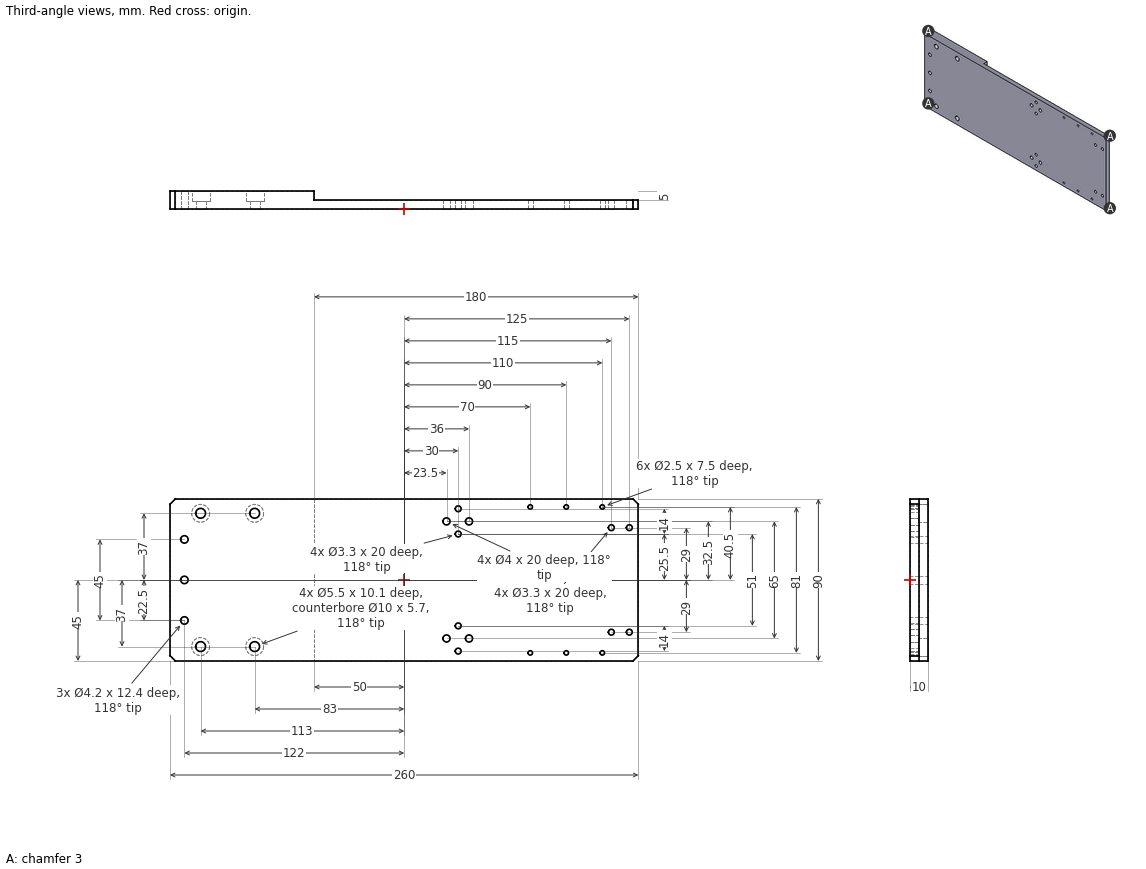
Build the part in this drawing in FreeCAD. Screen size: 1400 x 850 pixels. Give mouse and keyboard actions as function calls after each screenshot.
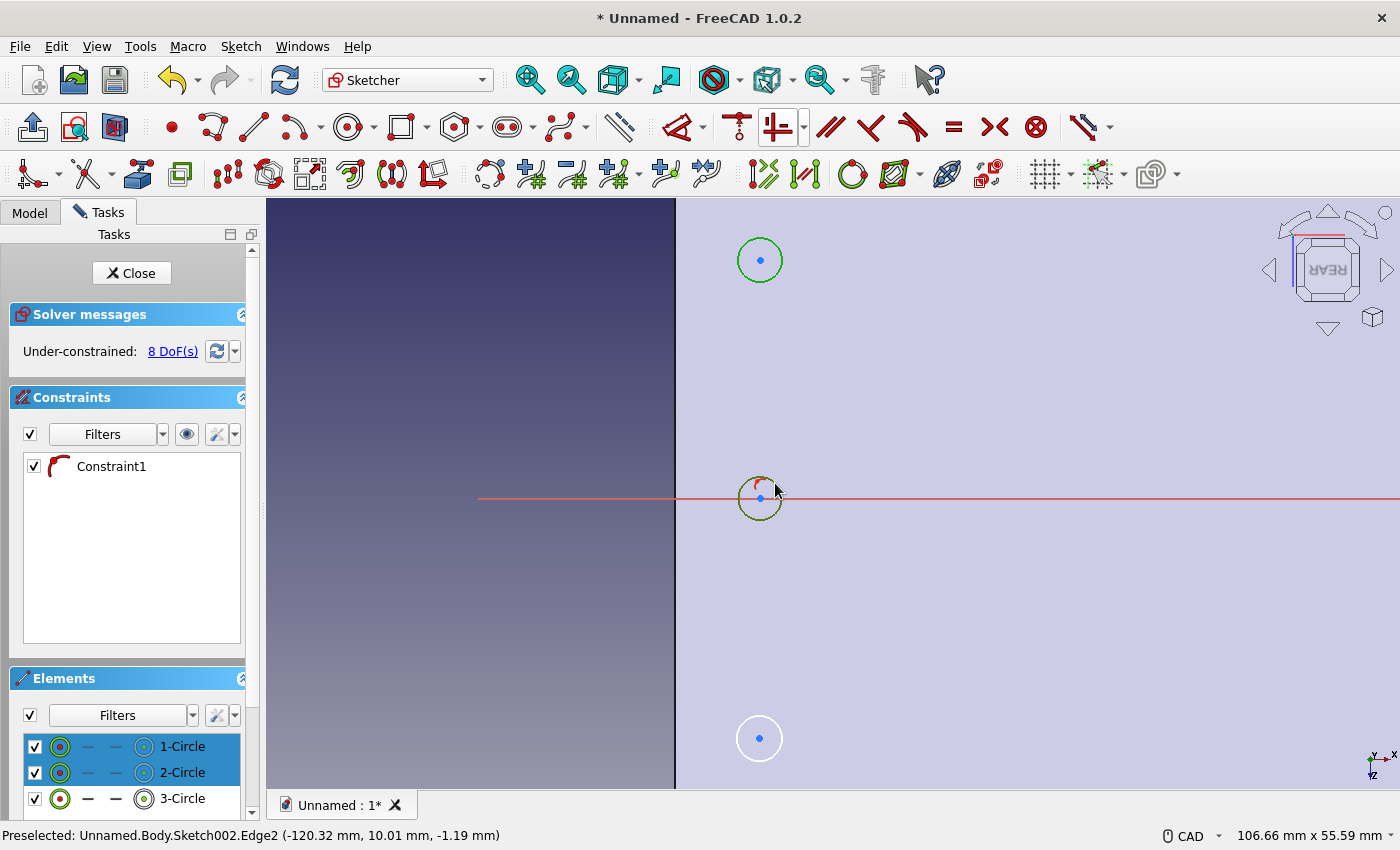
click(775, 723)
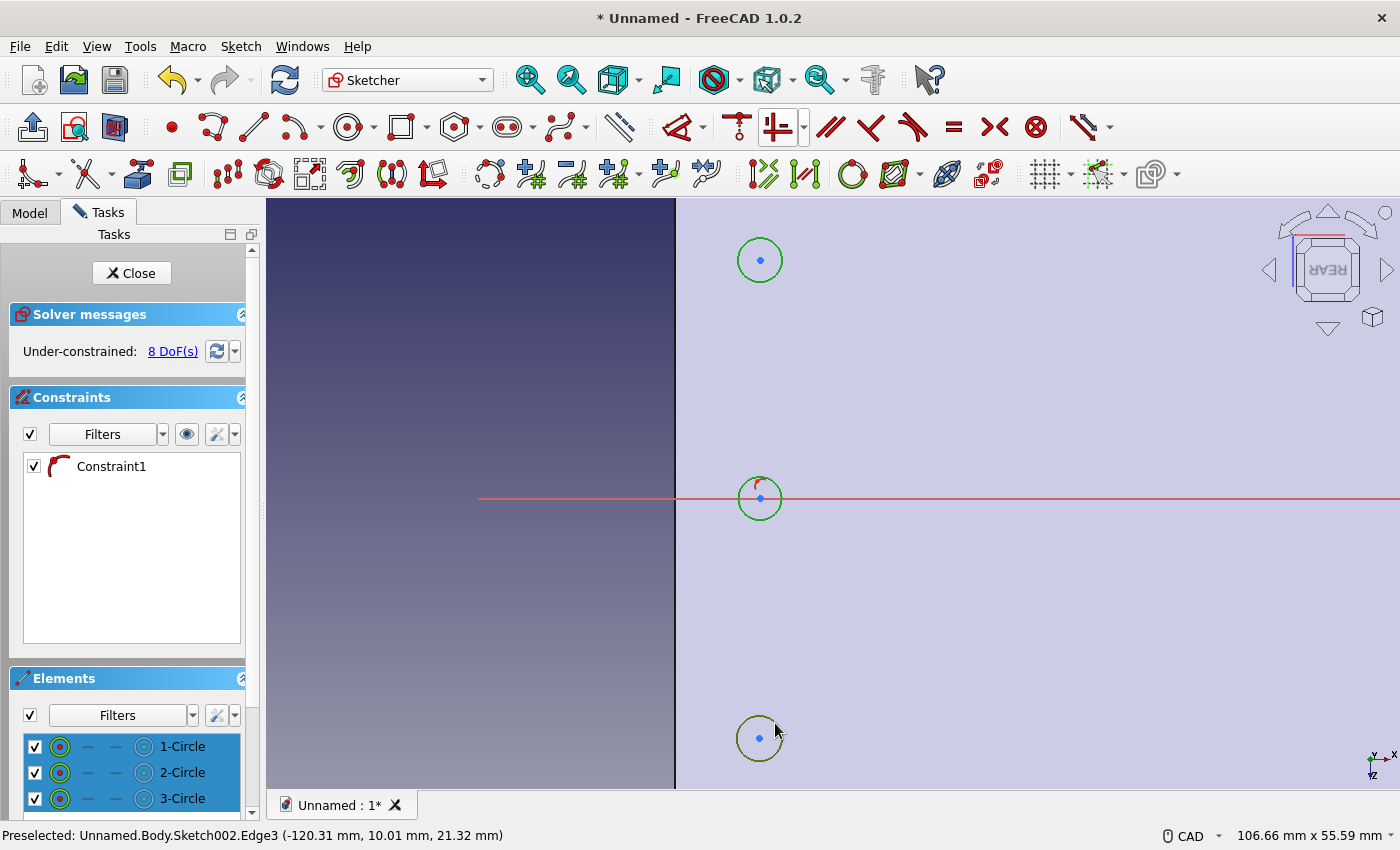
click(954, 128)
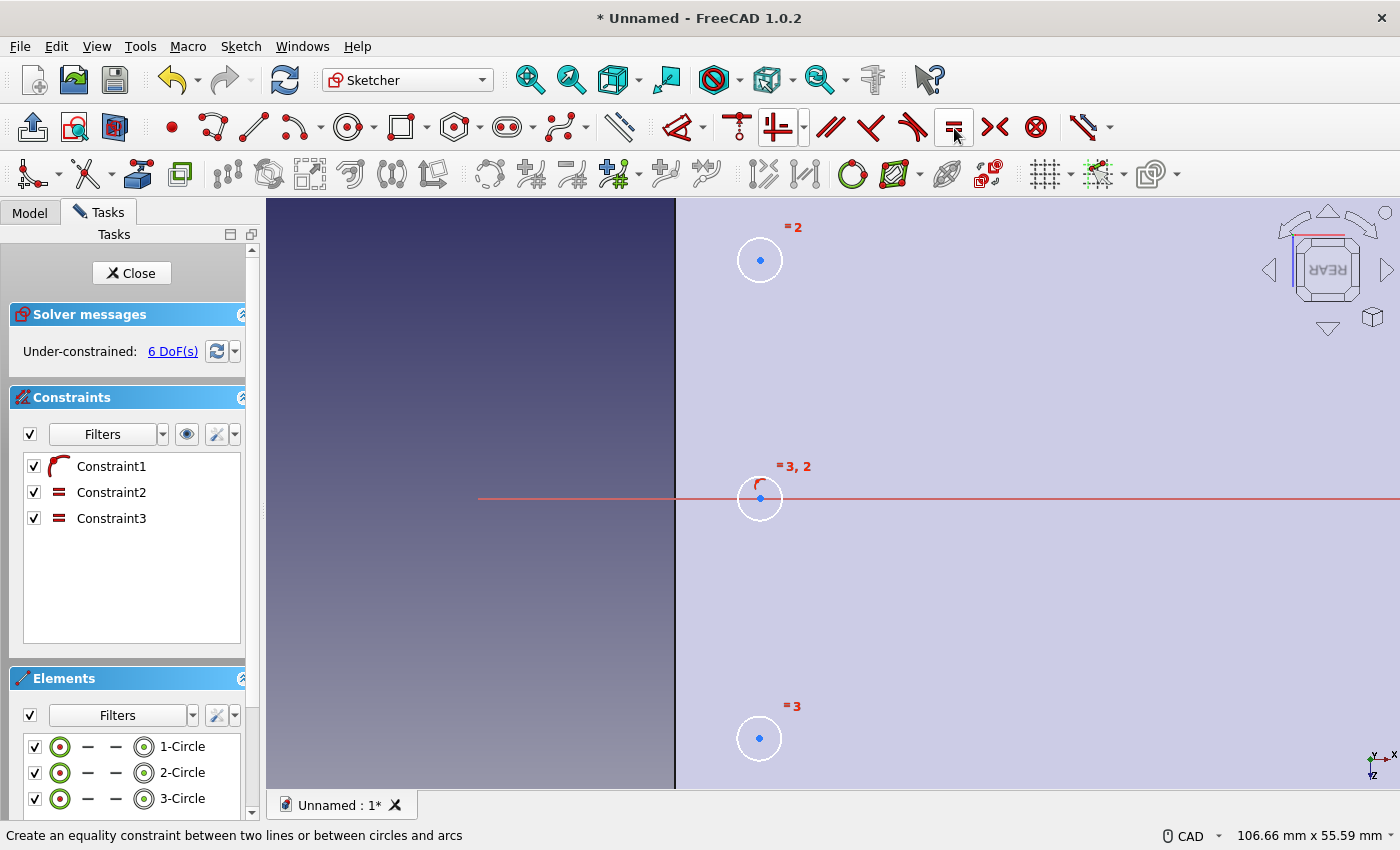
click(760, 260)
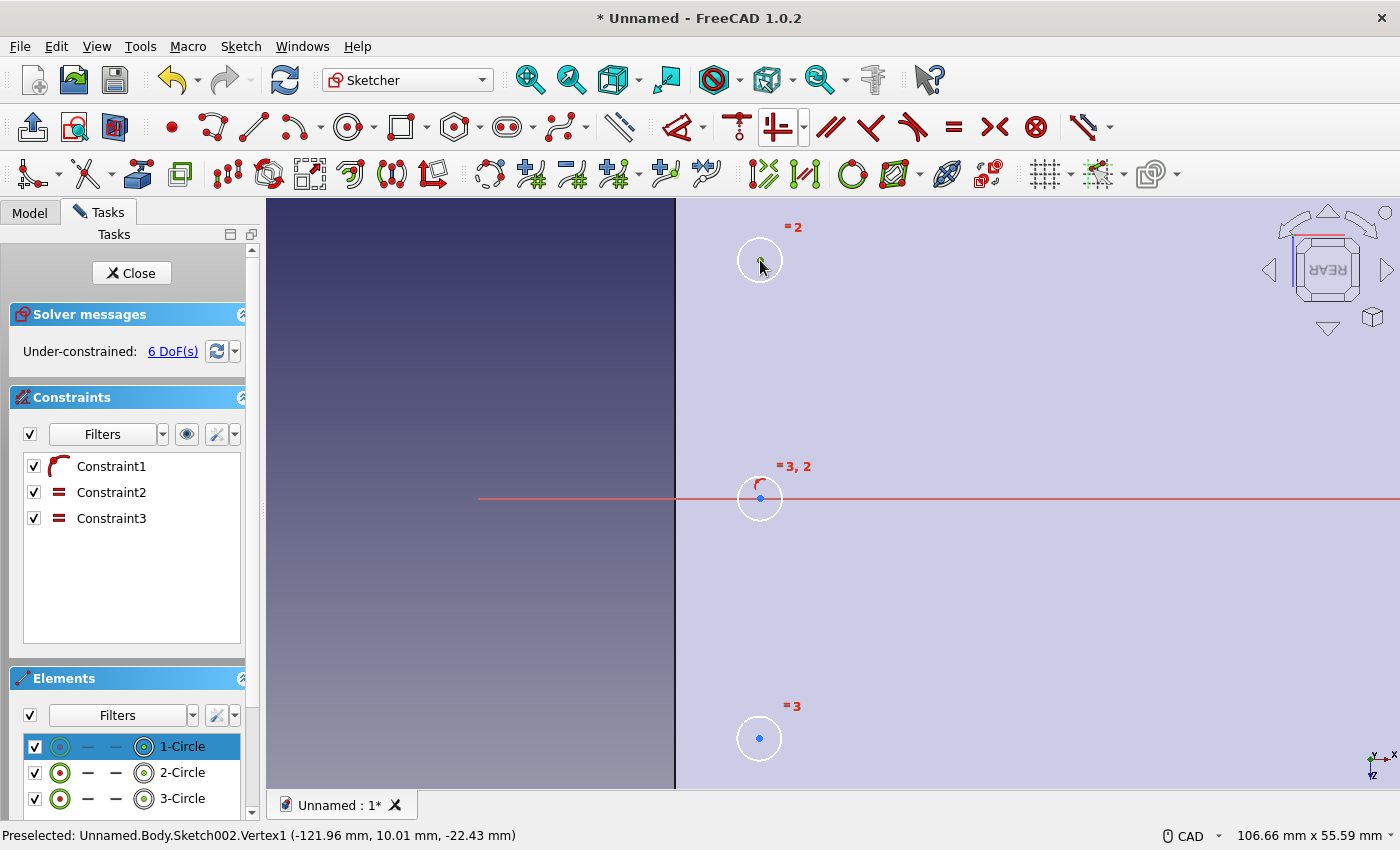
click(760, 499)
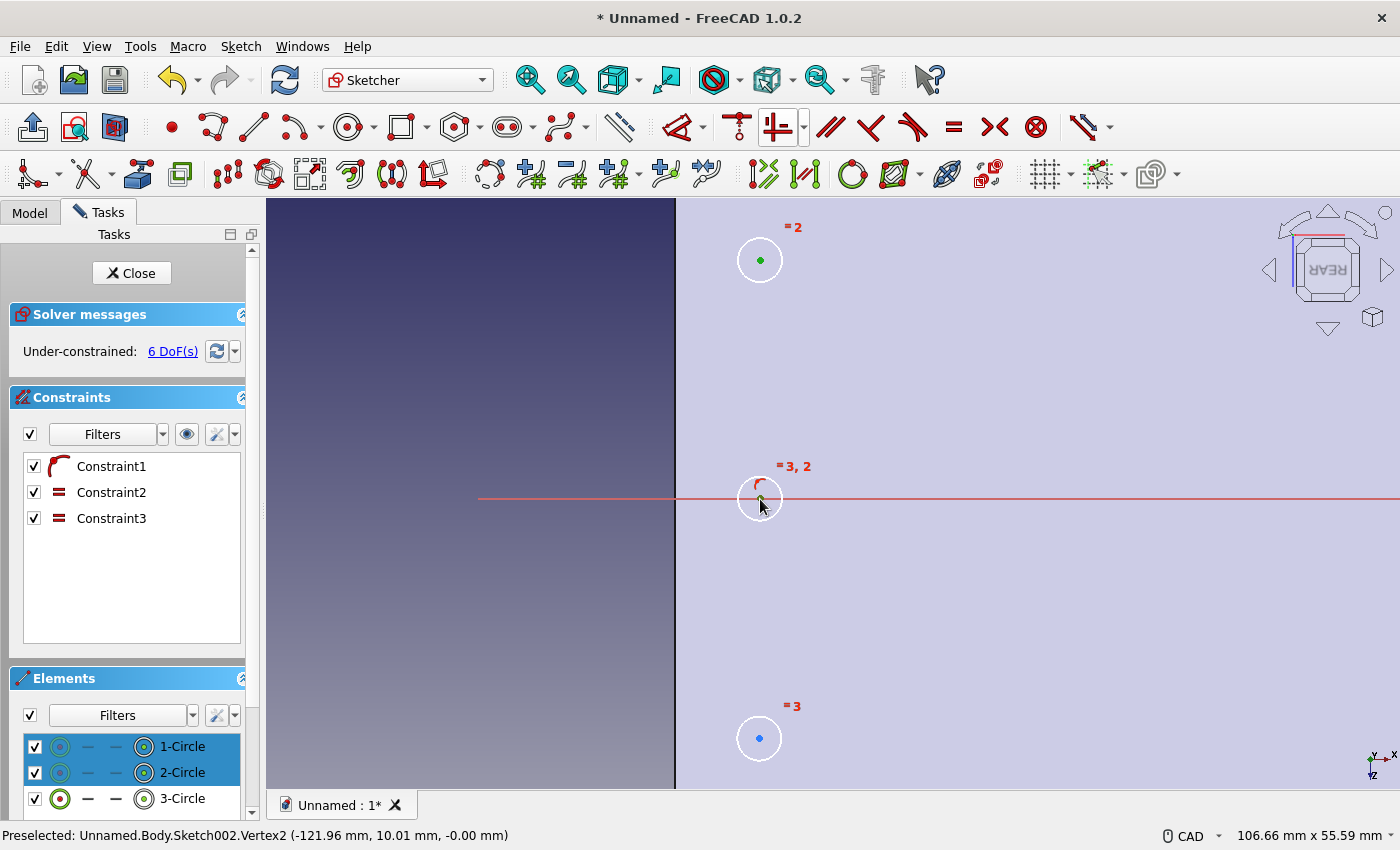
key(v)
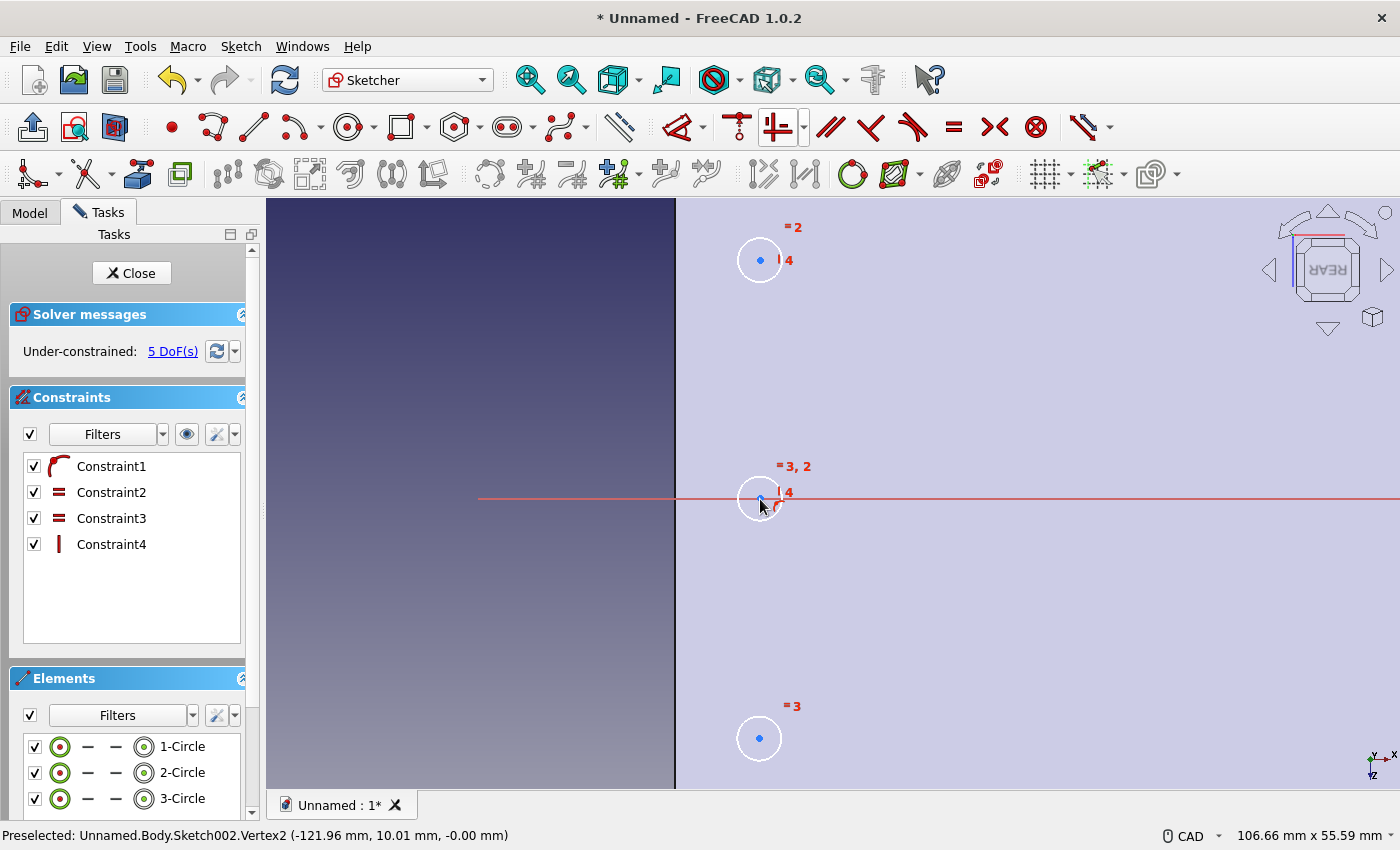
click(760, 499)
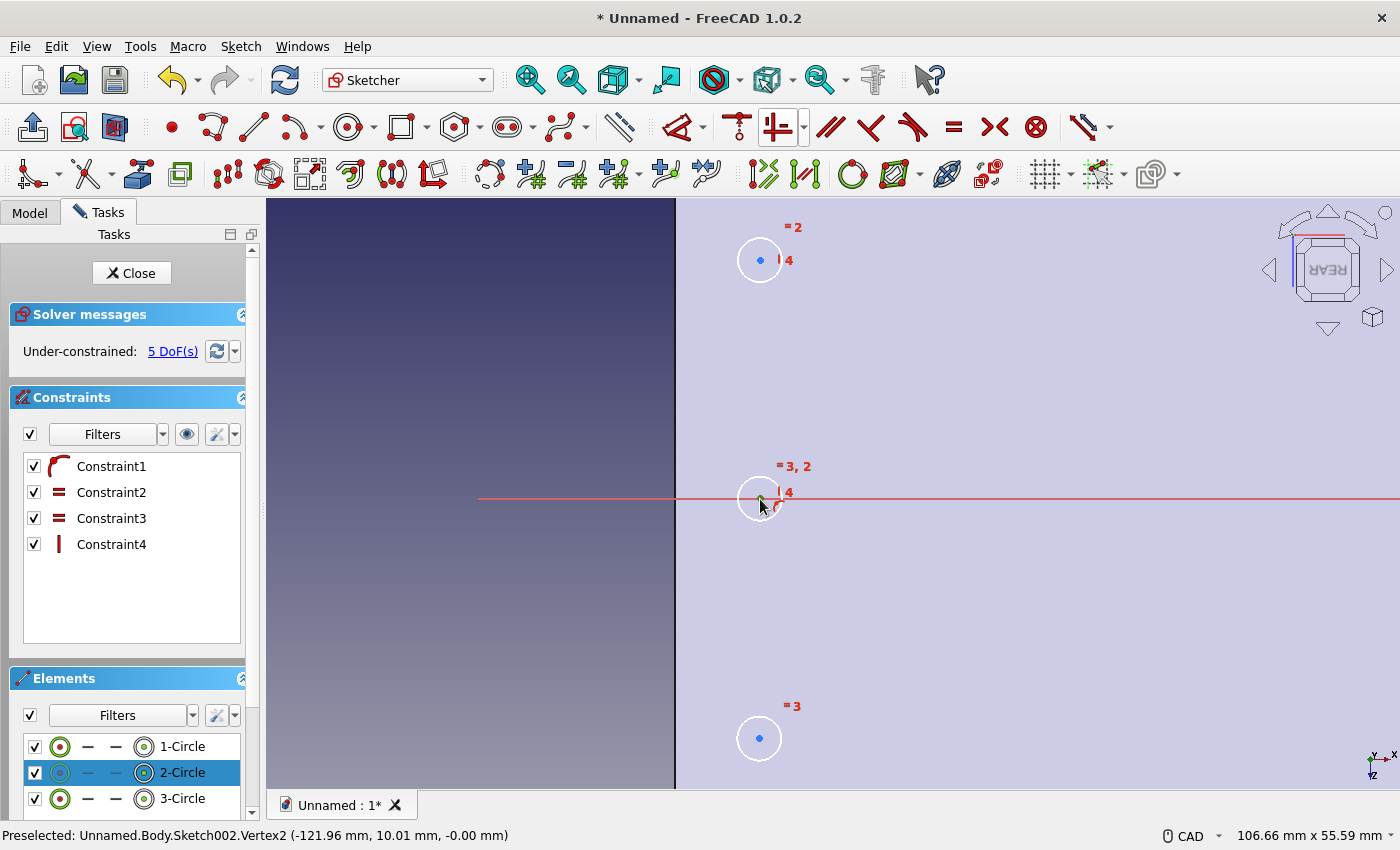
click(759, 739)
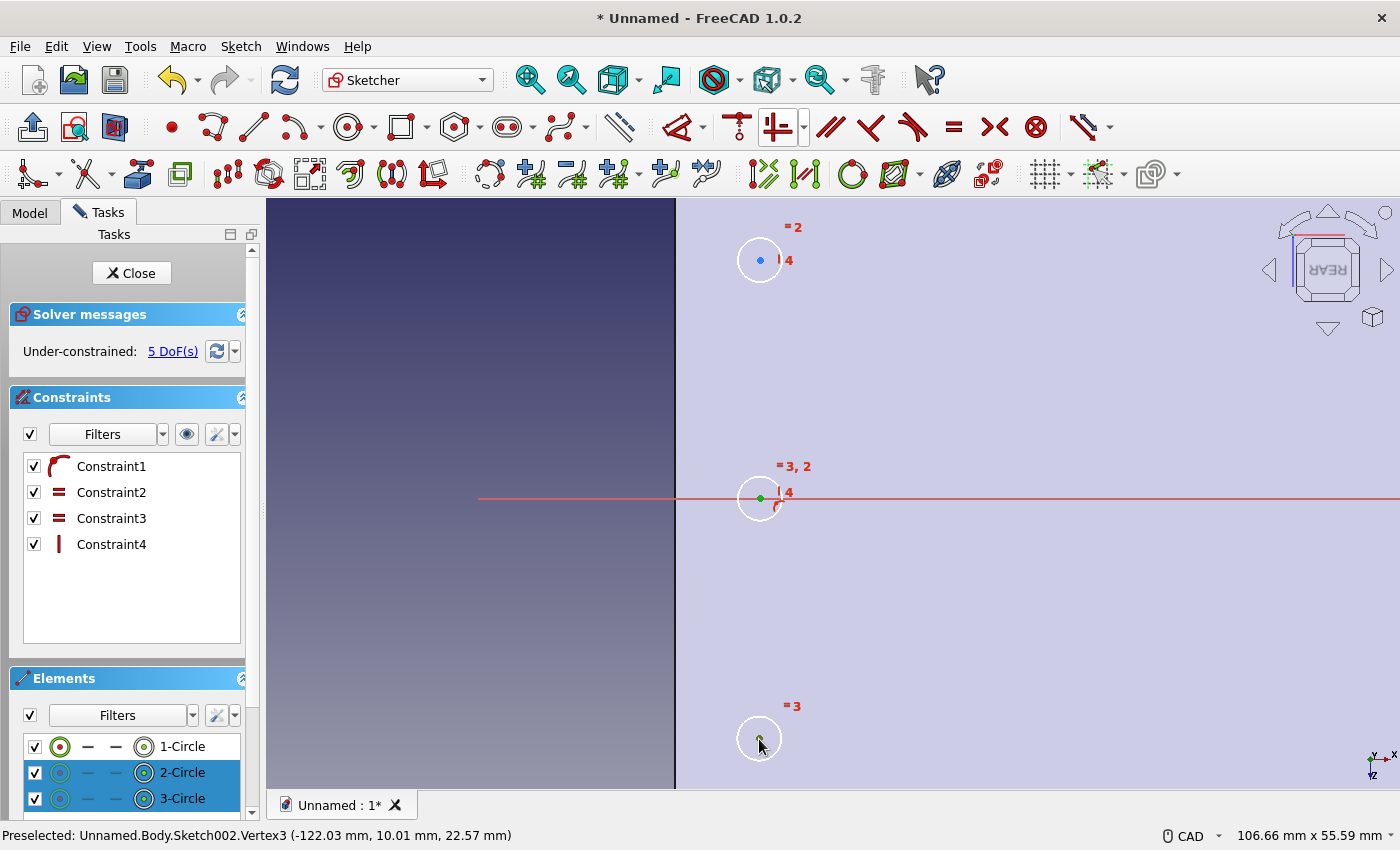
click(804, 128)